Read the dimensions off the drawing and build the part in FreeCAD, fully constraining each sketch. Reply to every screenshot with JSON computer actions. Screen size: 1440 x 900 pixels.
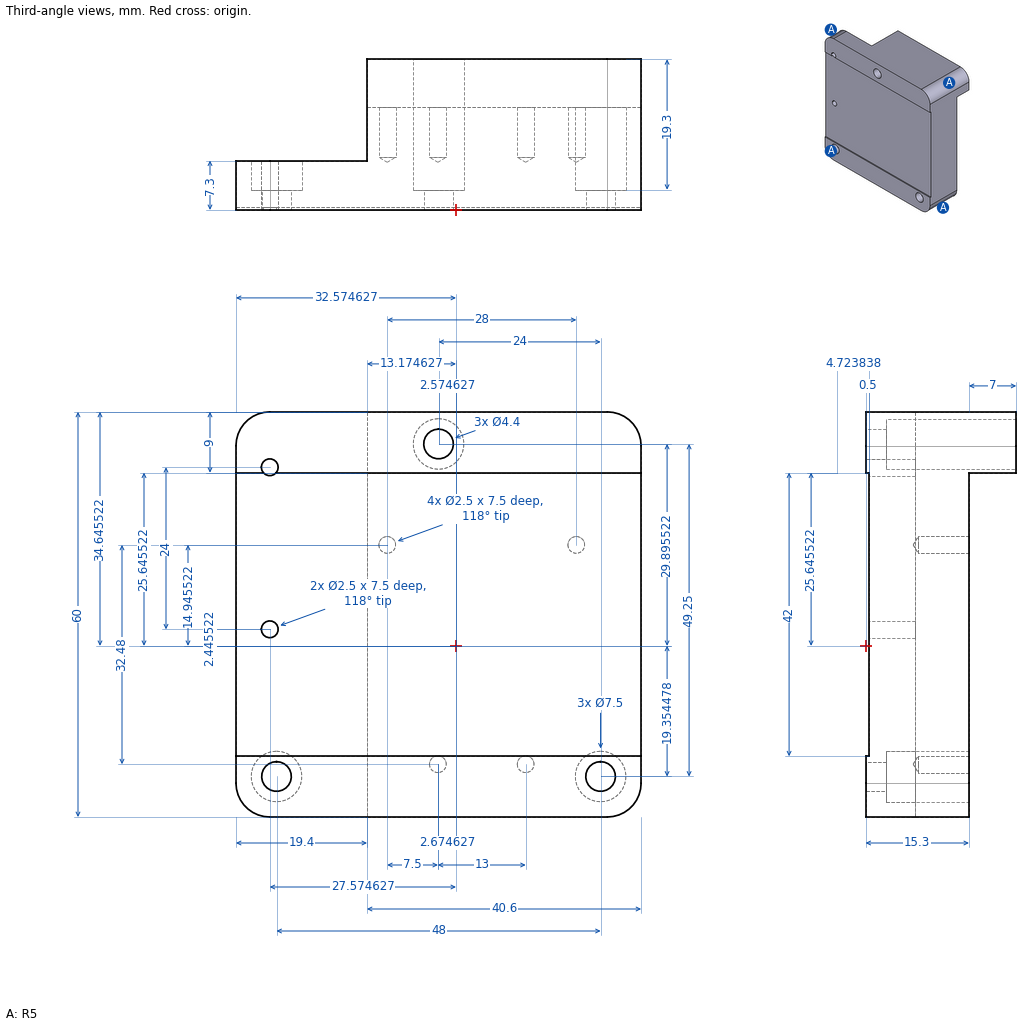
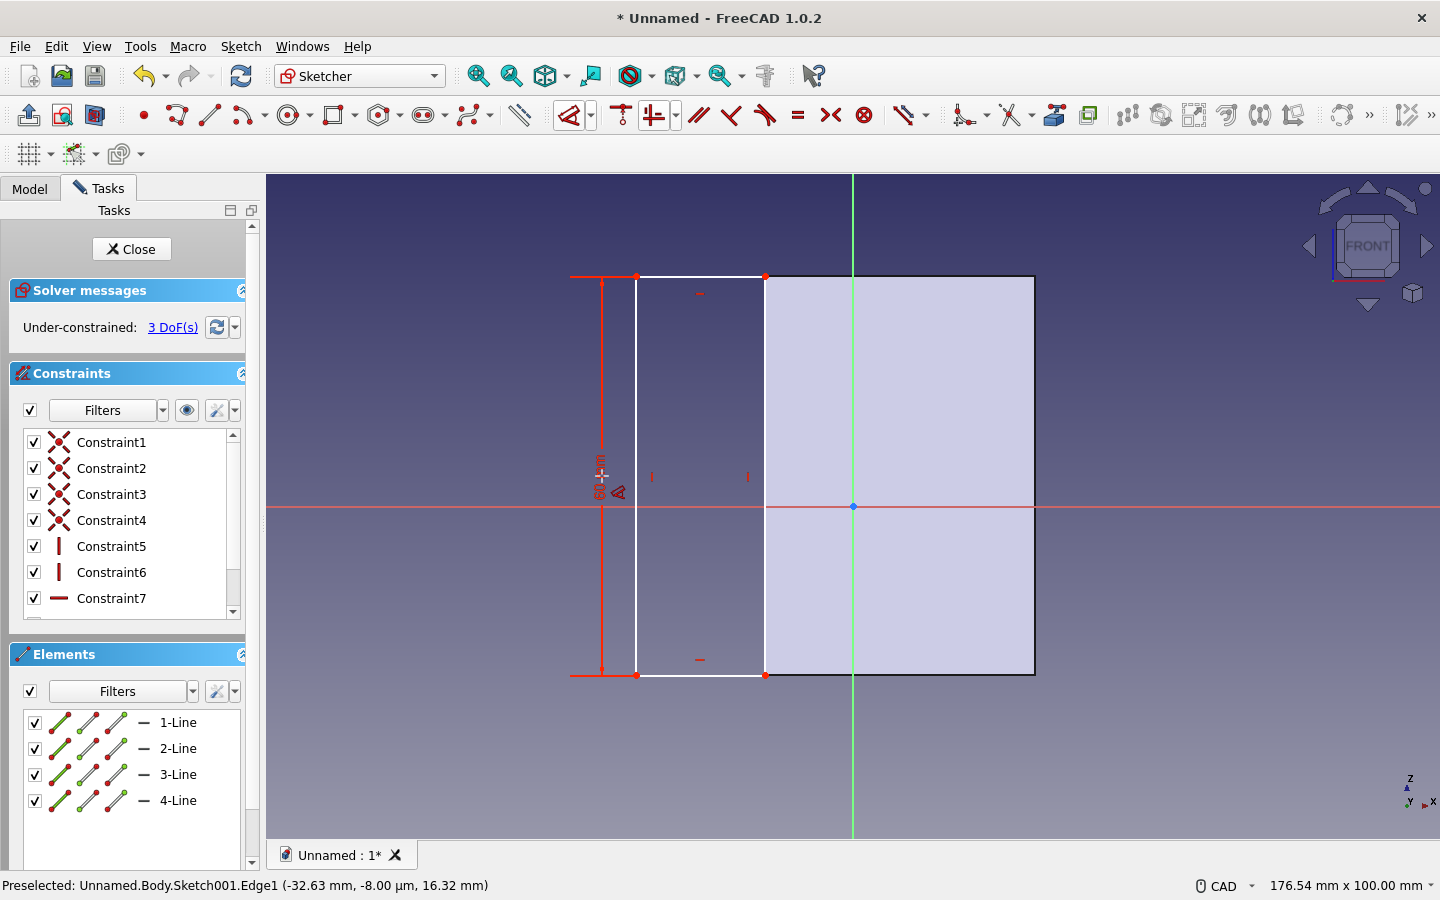
{"action": "left_click", "coordinate": [675, 676]}
{"action": "left_click", "coordinate": [701, 710]}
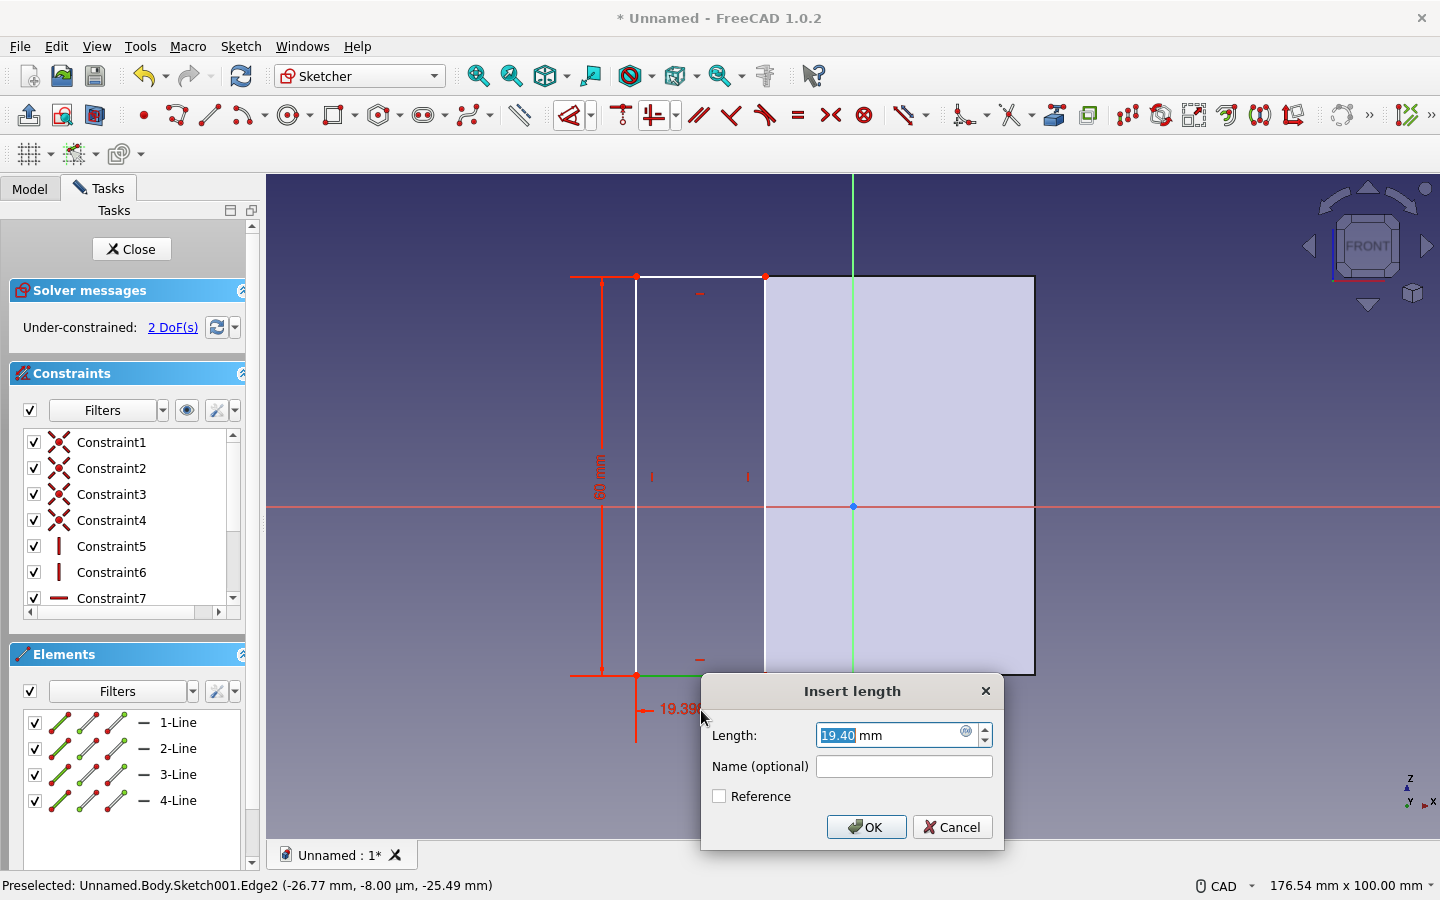
{"action": "type", "text": "19.4"}
{"action": "key", "text": "Return"}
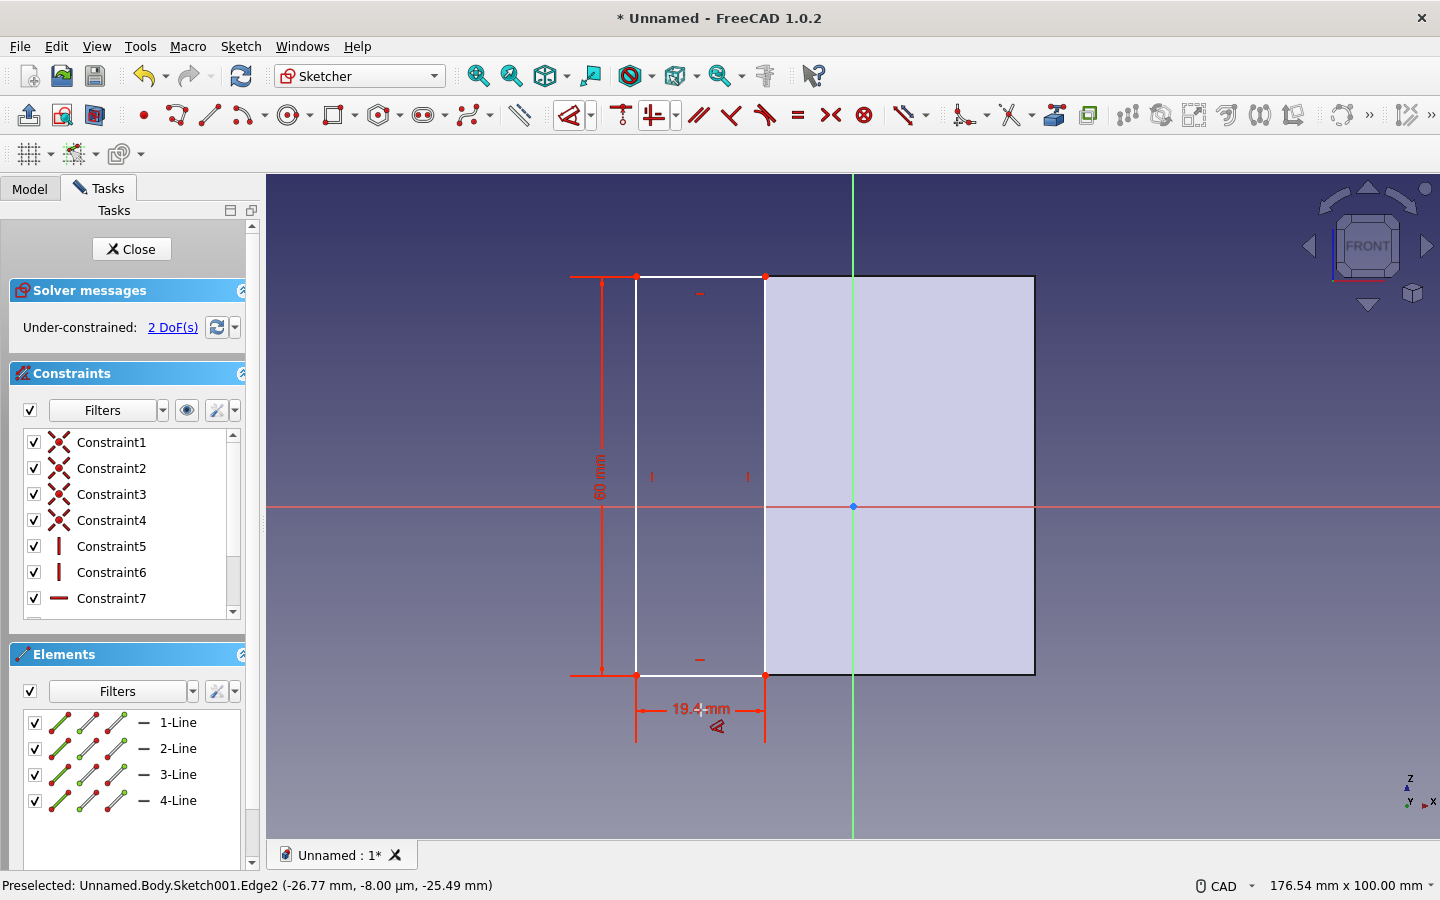
{"action": "left_click", "coordinate": [636, 277]}
{"action": "left_click", "coordinate": [744, 243]}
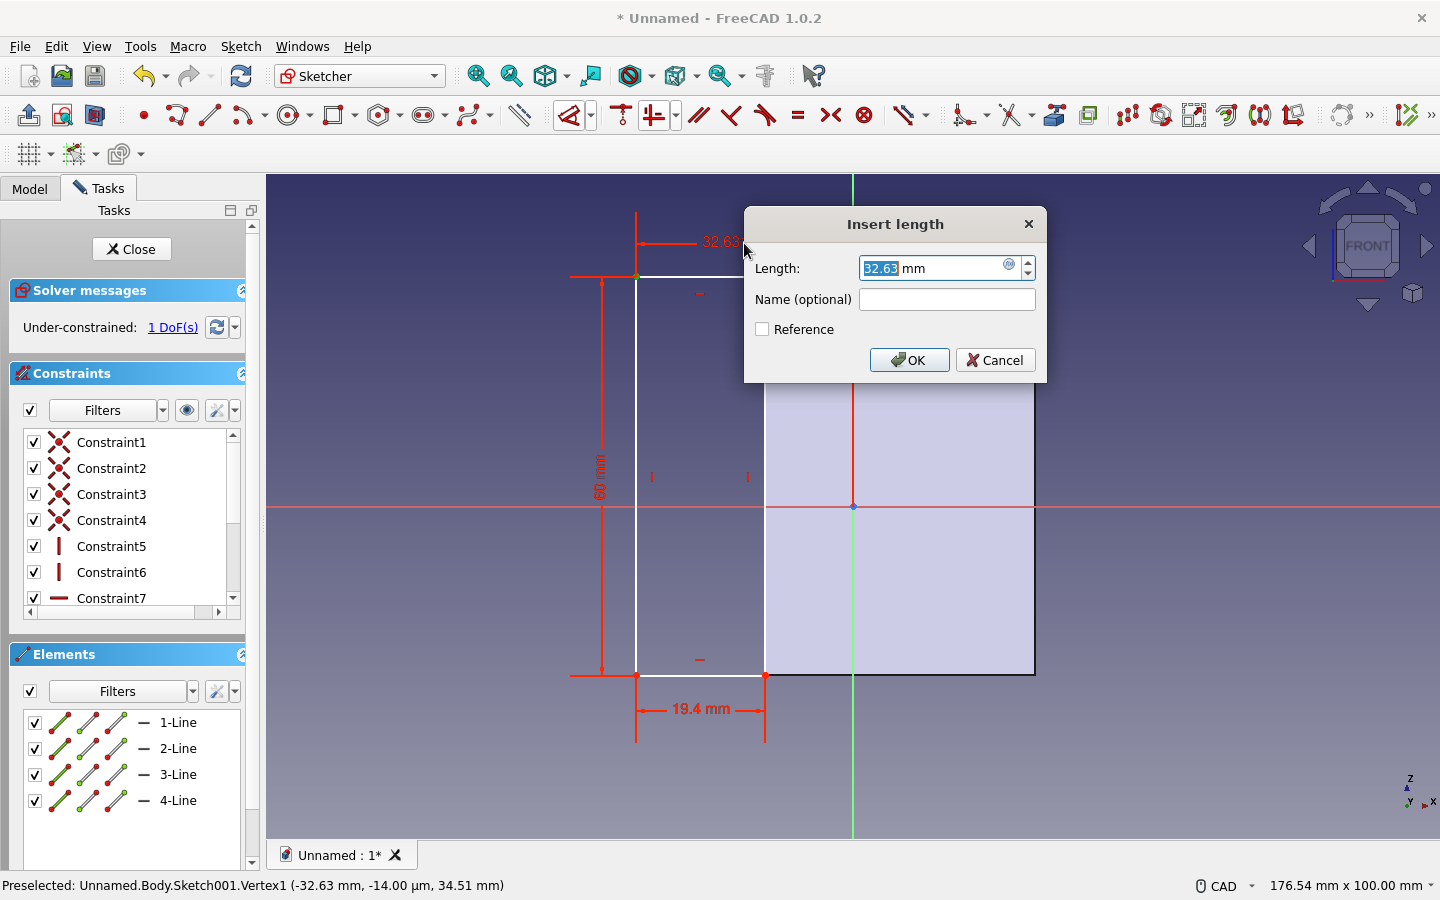
{"action": "type", "text": "32.574627"}
{"action": "key", "text": "Return"}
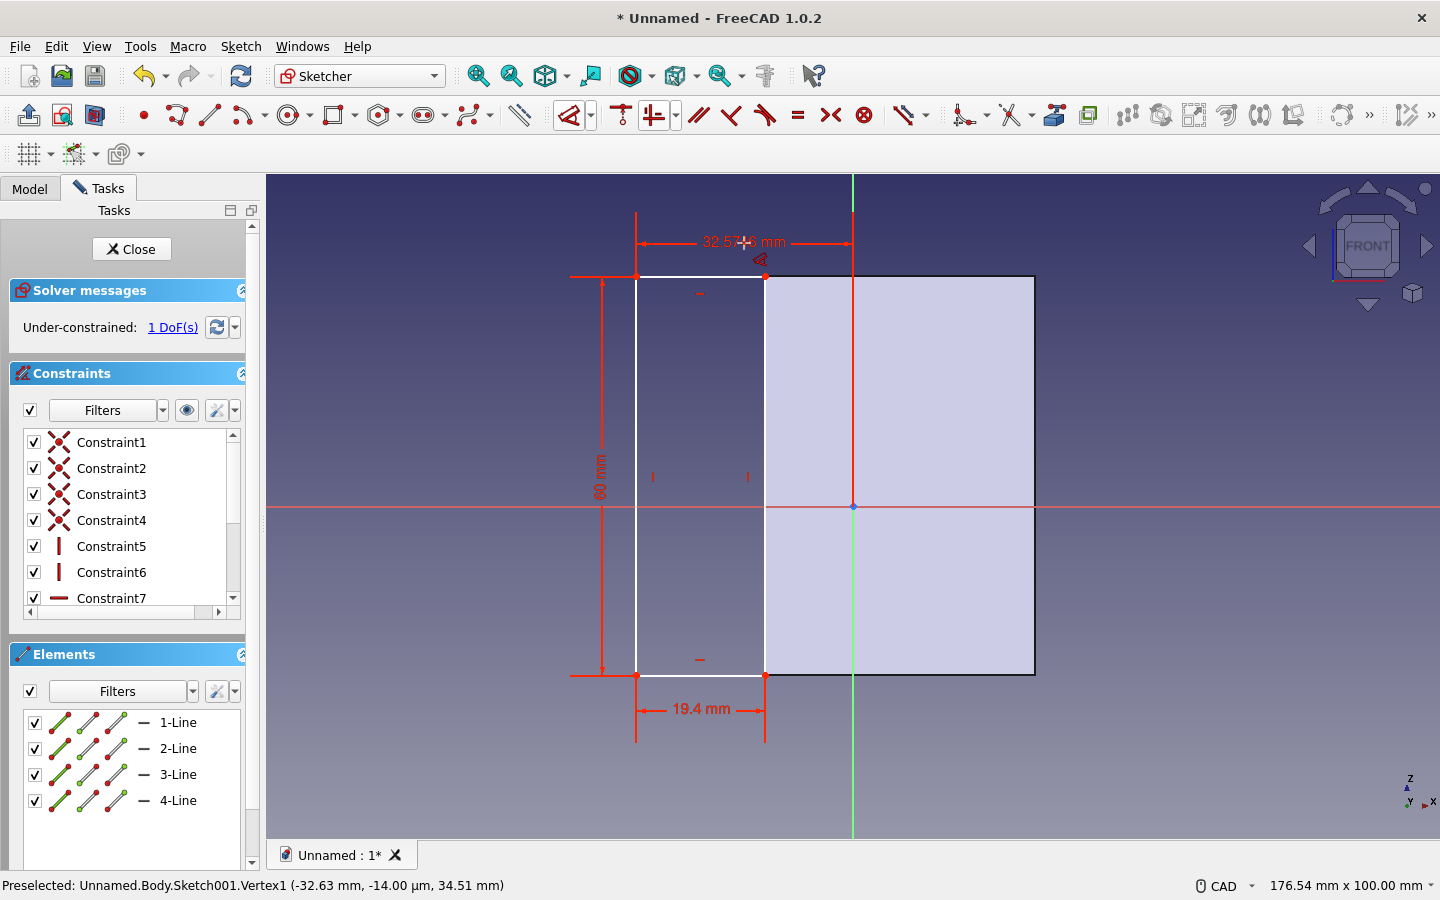
{"action": "left_click", "coordinate": [636, 277]}
{"action": "left_click", "coordinate": [602, 392]}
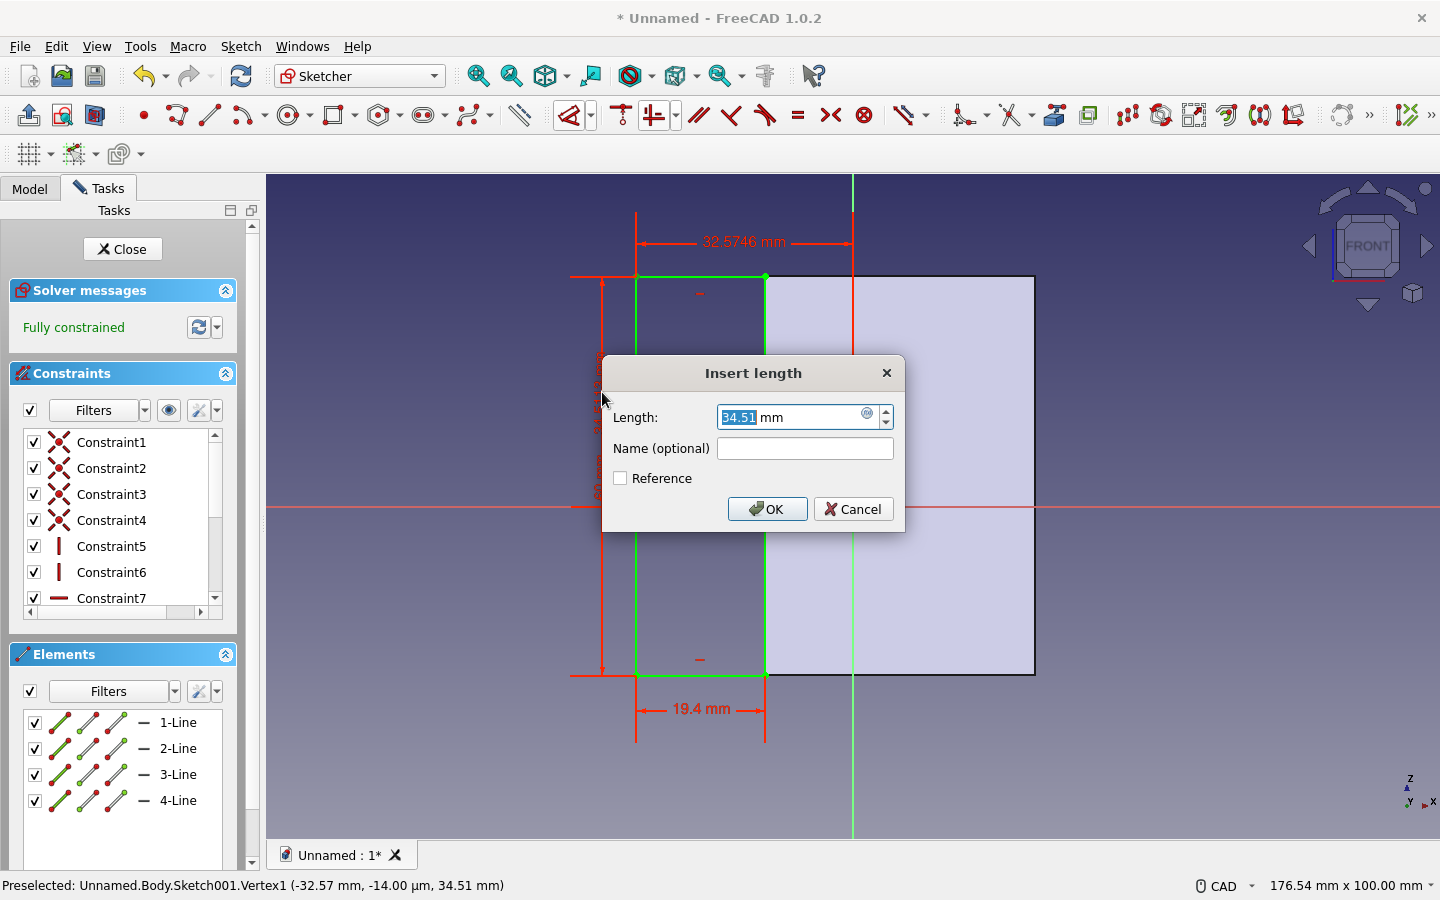
{"action": "type", "text": "34.645522"}
{"action": "key", "text": "Return"}
{"action": "key", "text": "Escape"}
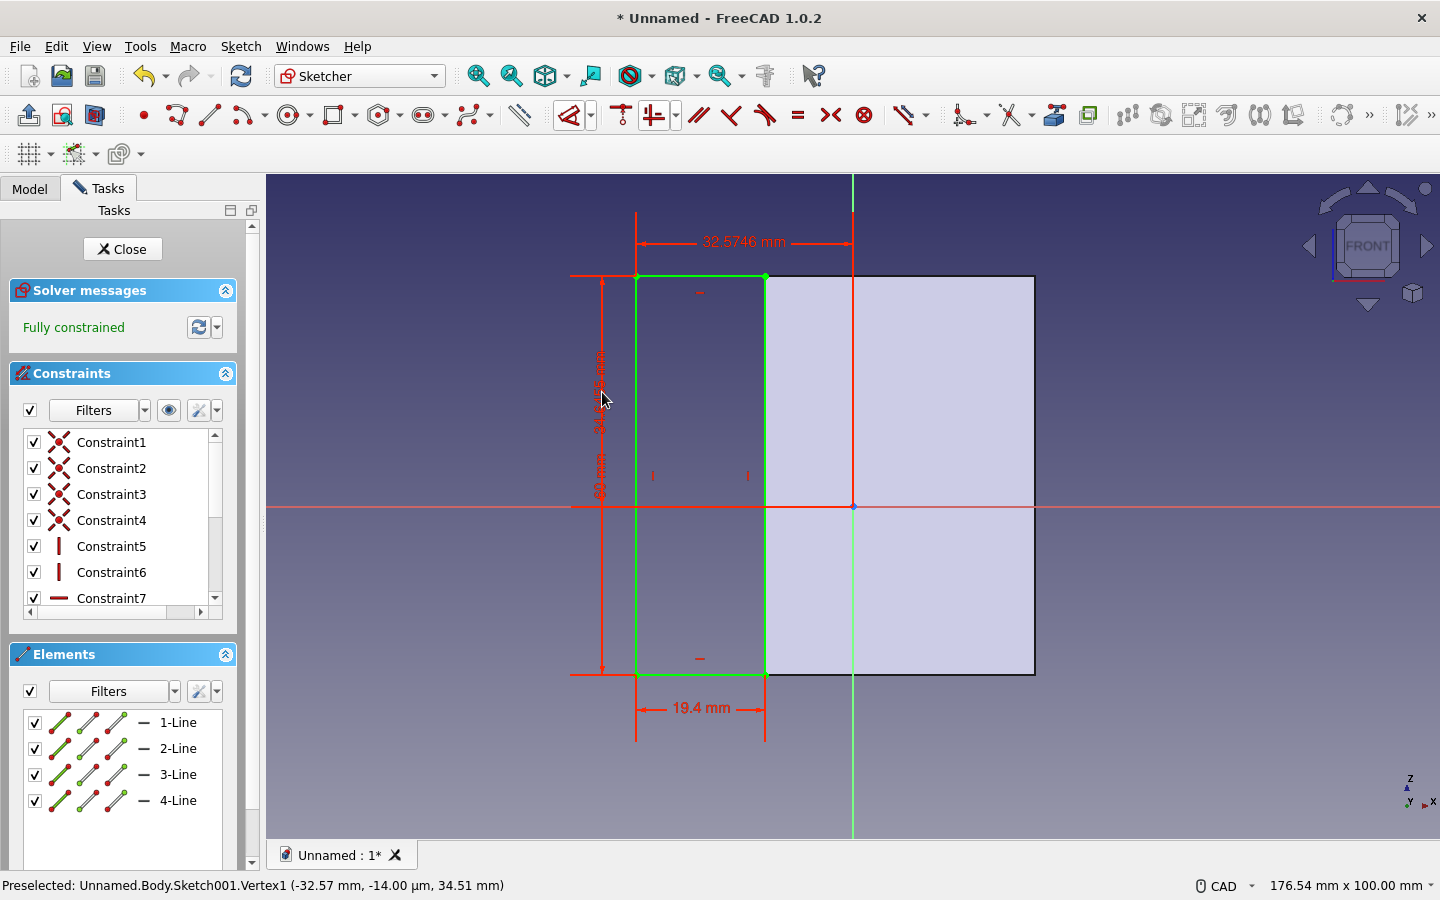
{"action": "left_click", "coordinate": [123, 249]}